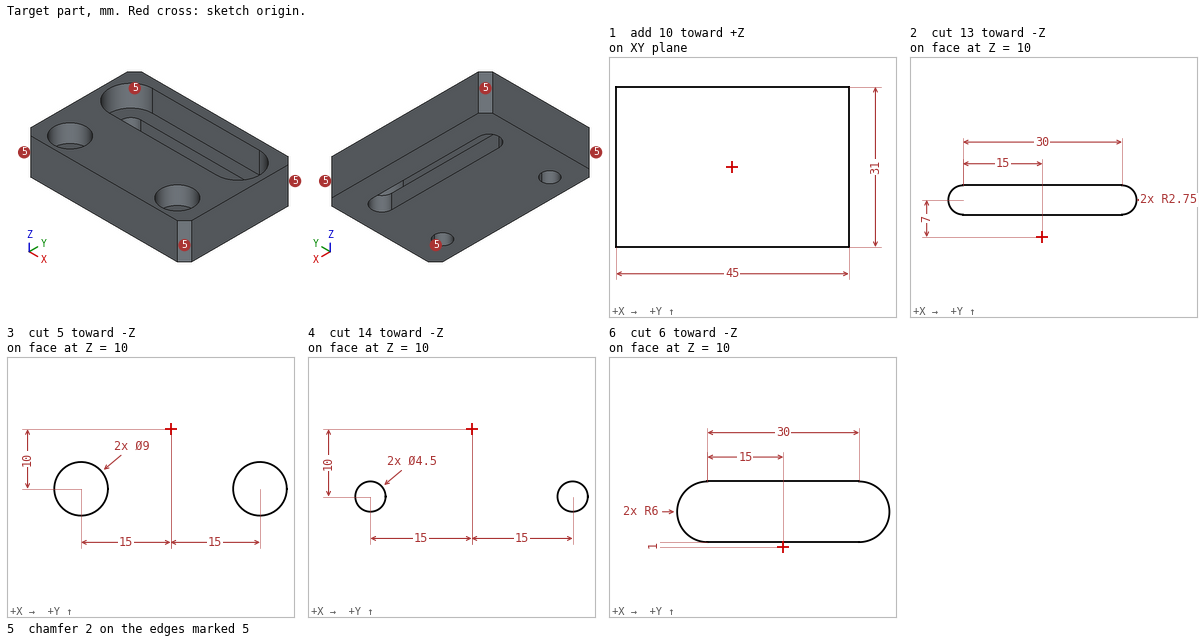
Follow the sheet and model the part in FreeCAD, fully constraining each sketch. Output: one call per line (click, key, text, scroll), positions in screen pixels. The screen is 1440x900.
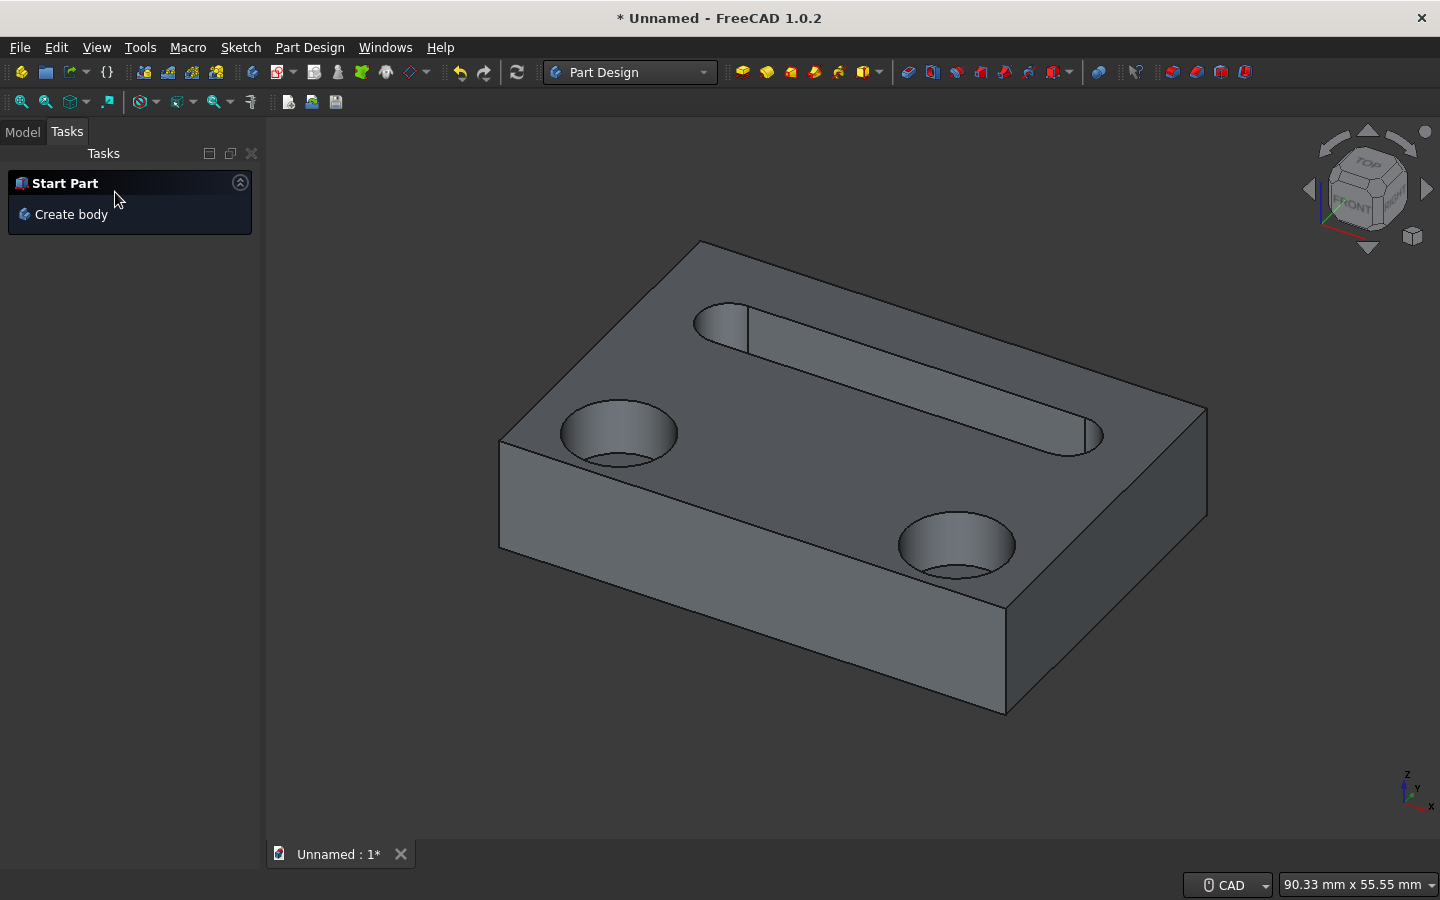
click(1006, 661)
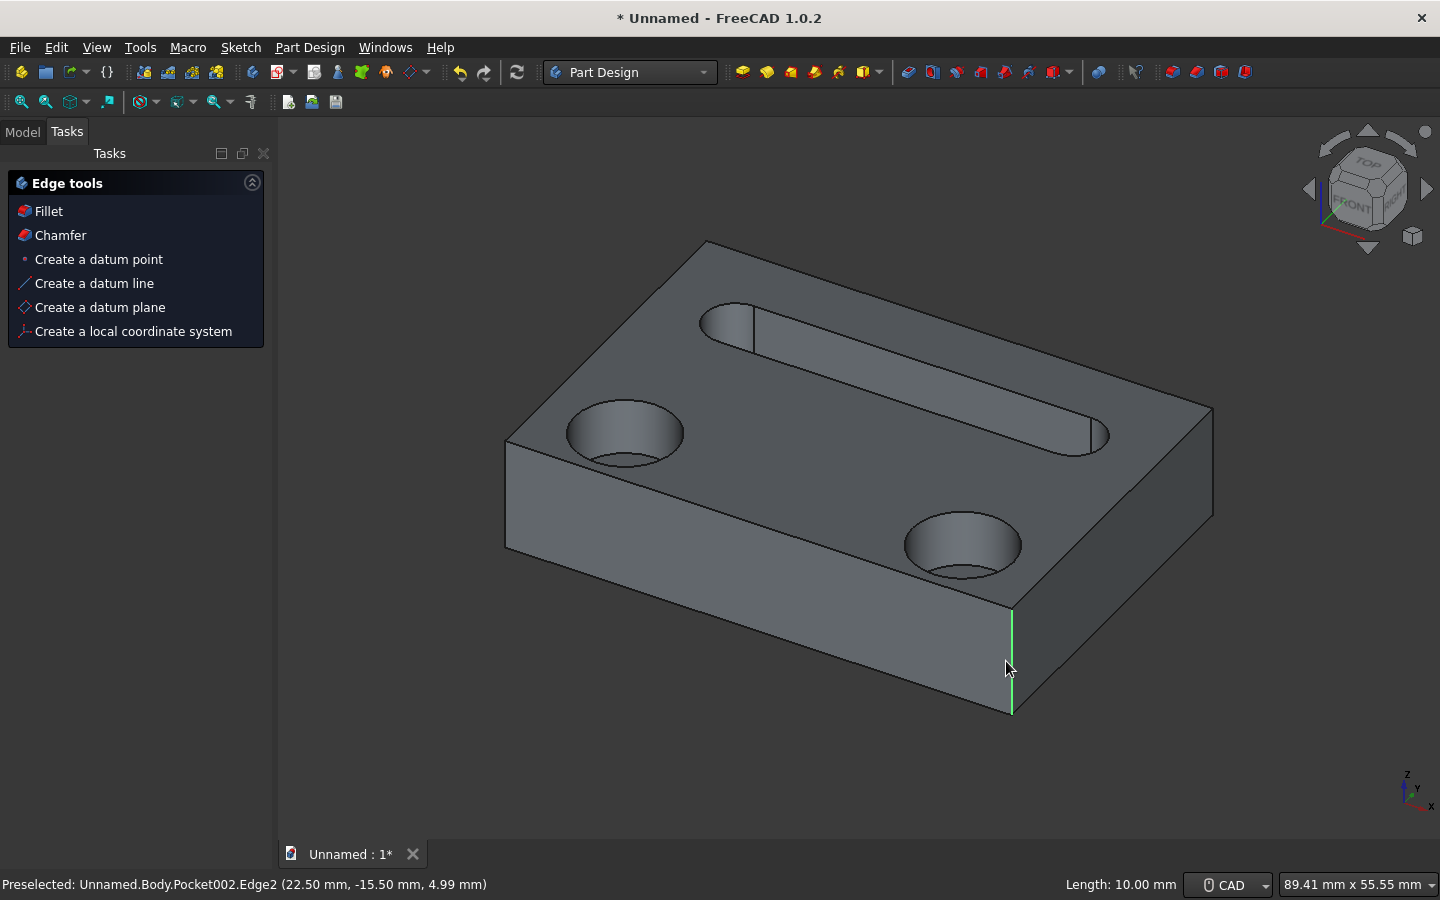
key(0)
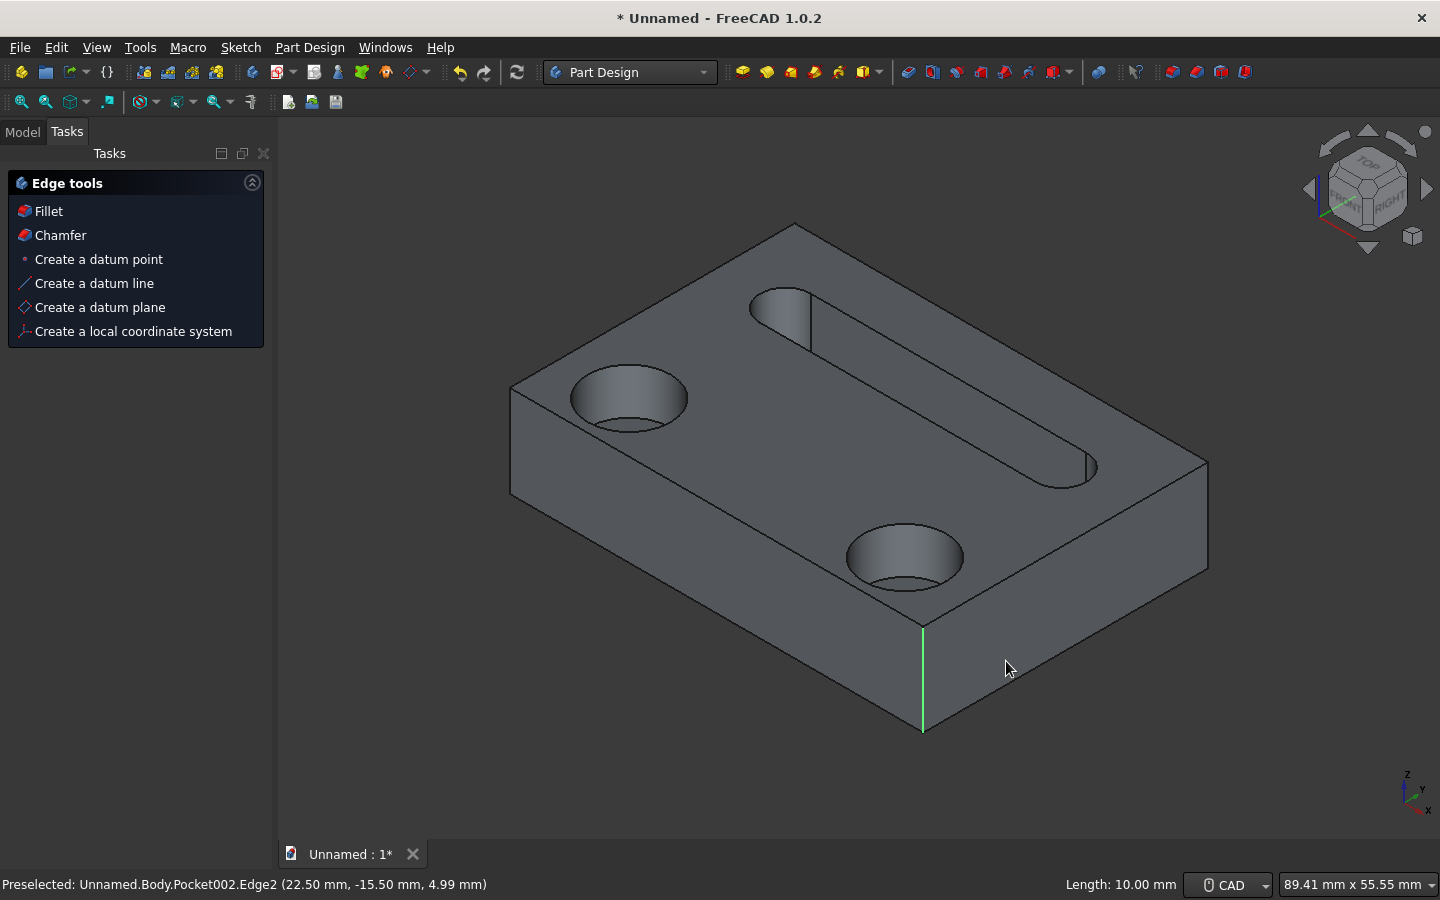
key(2)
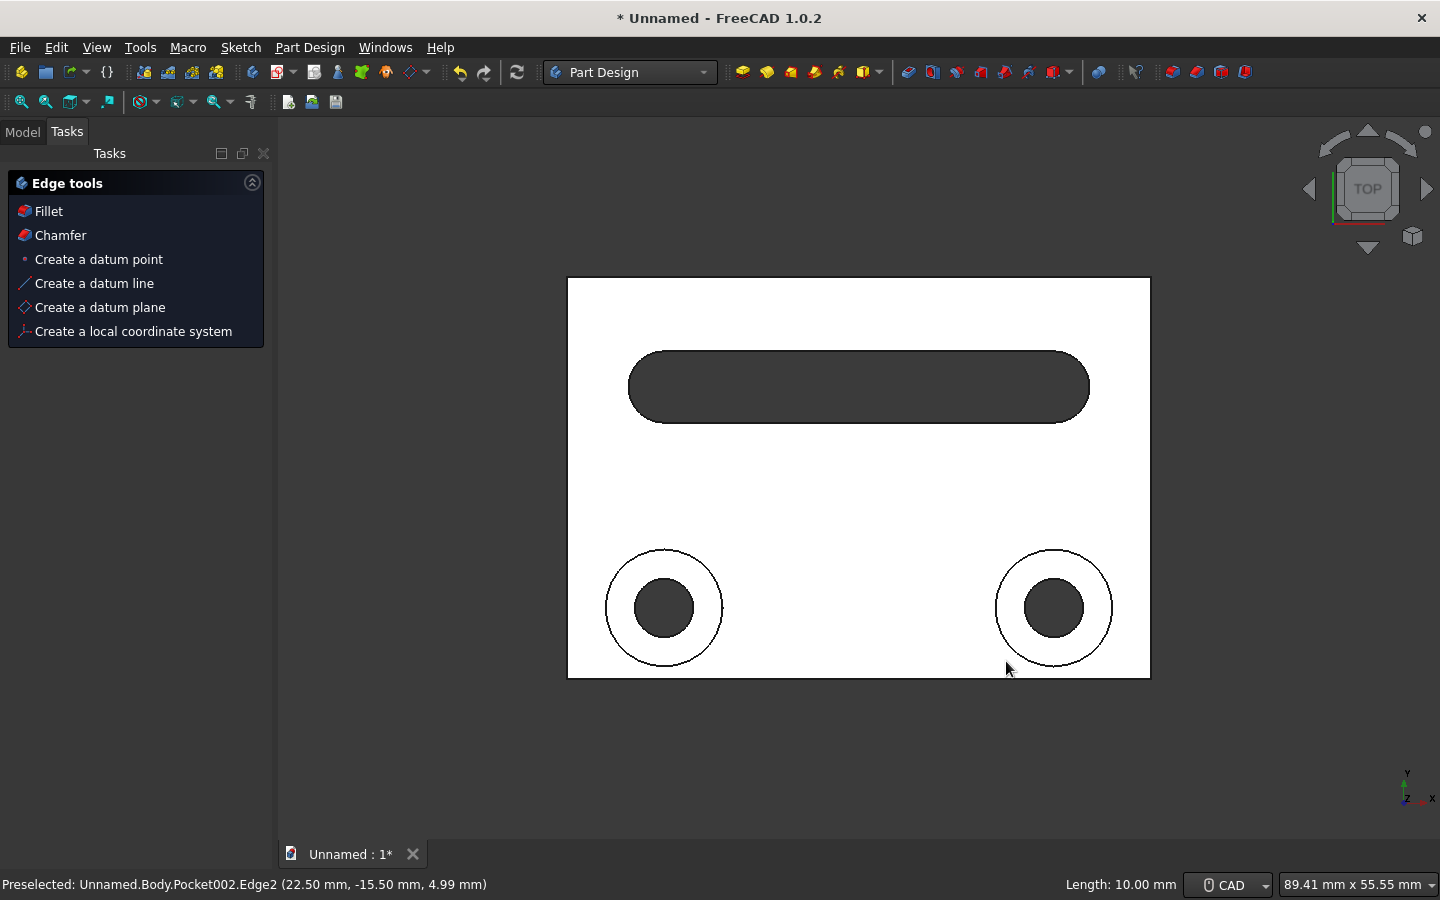
key(1)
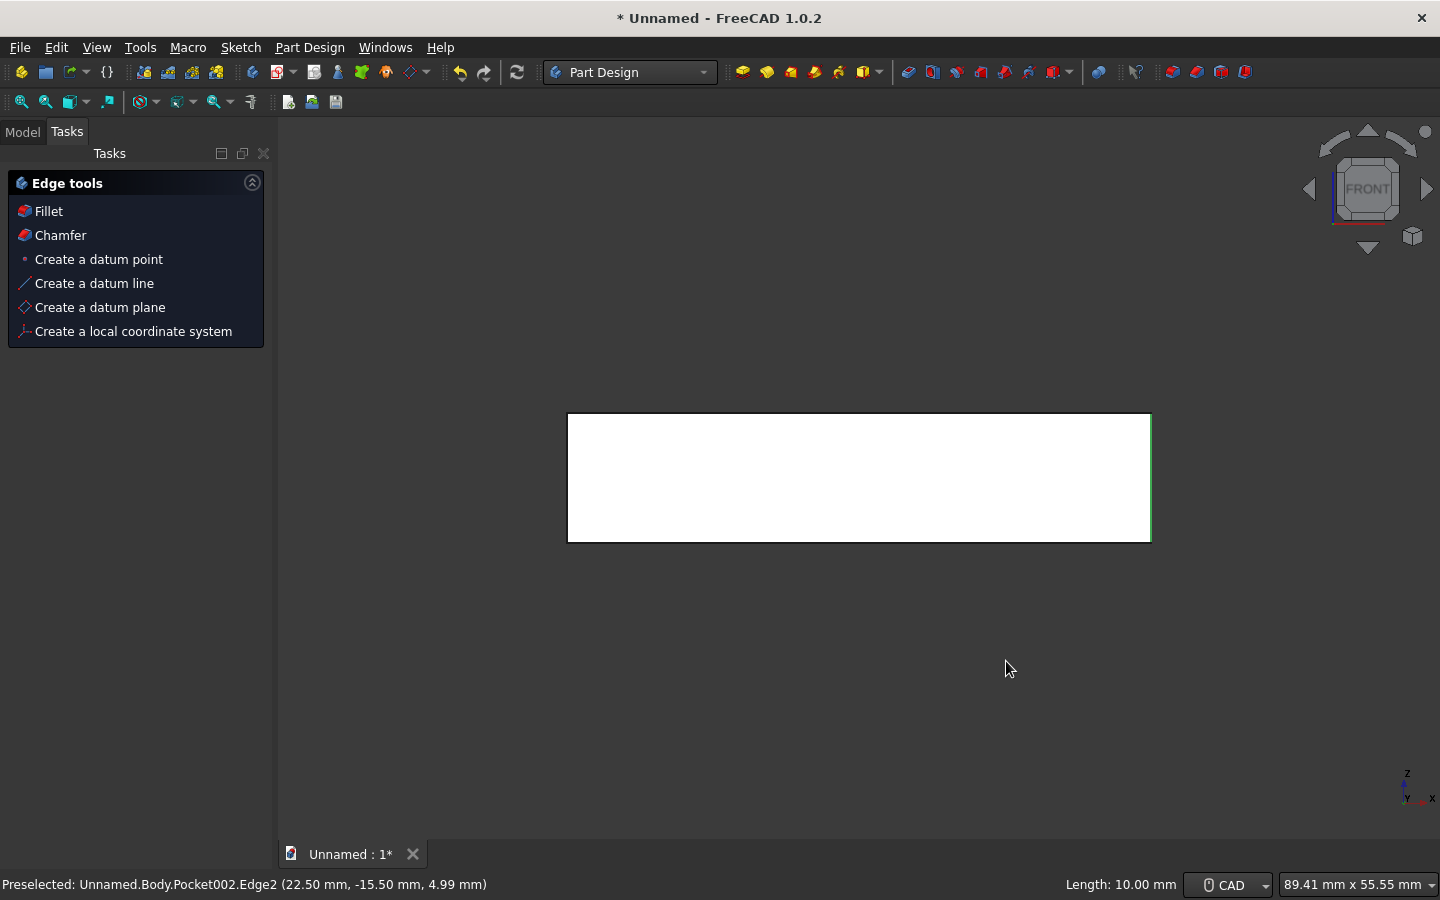
click(567, 477, ctrl)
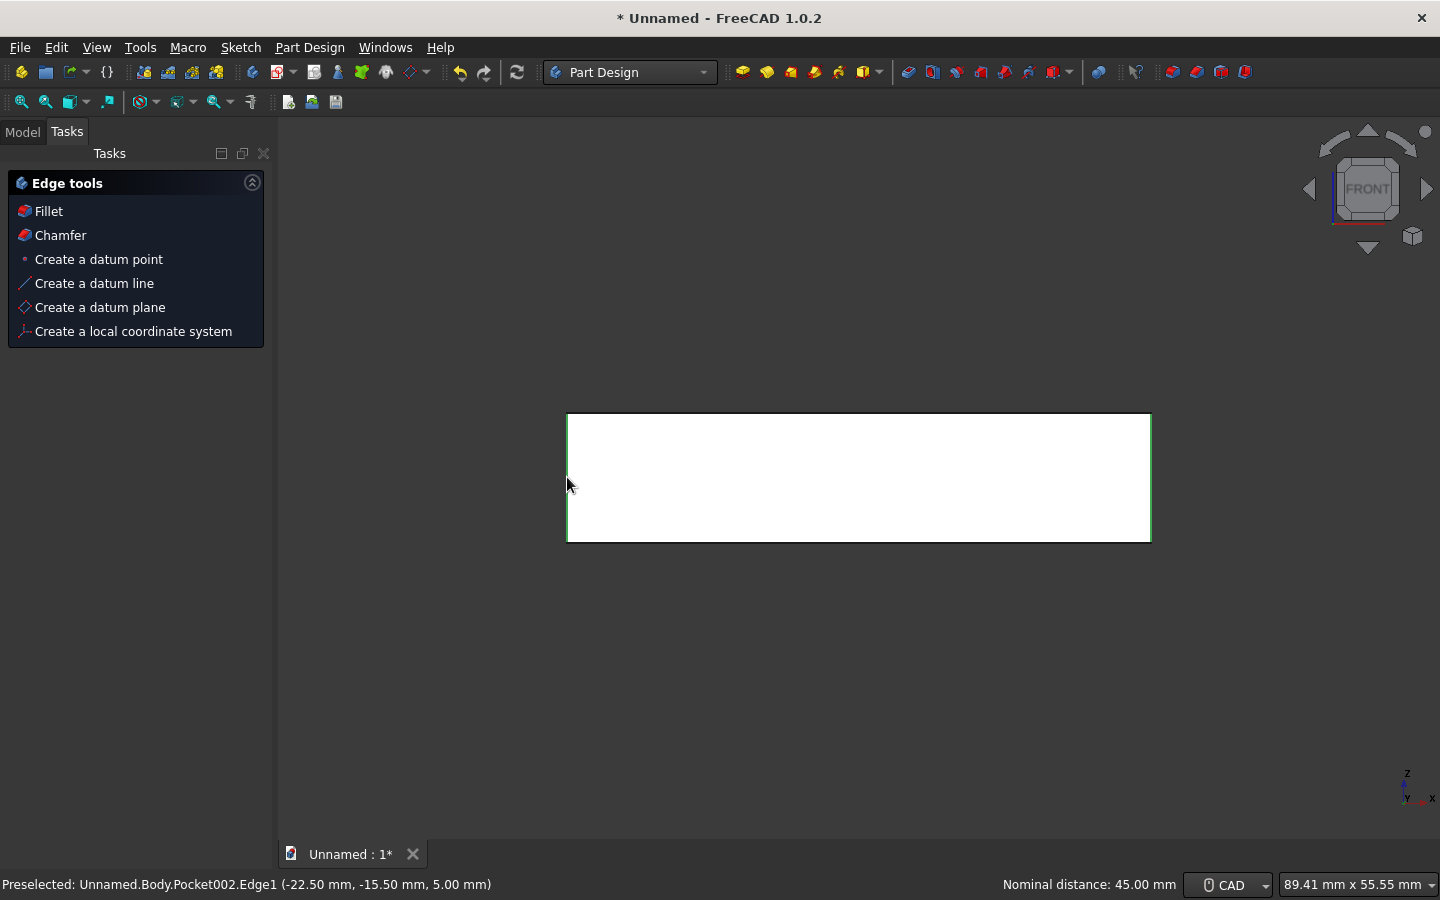
key(3)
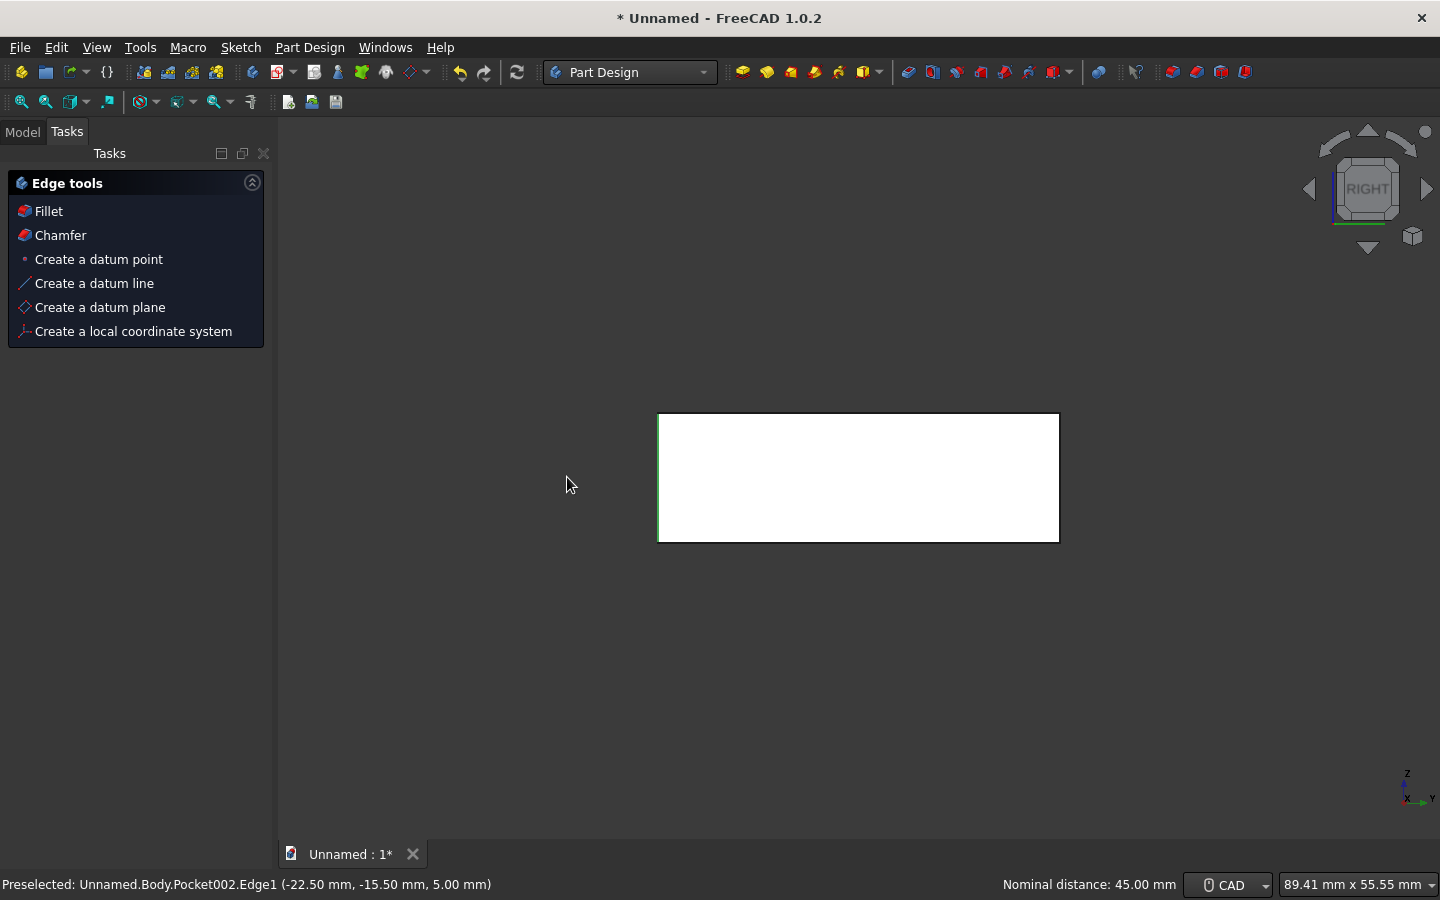
click(22, 102)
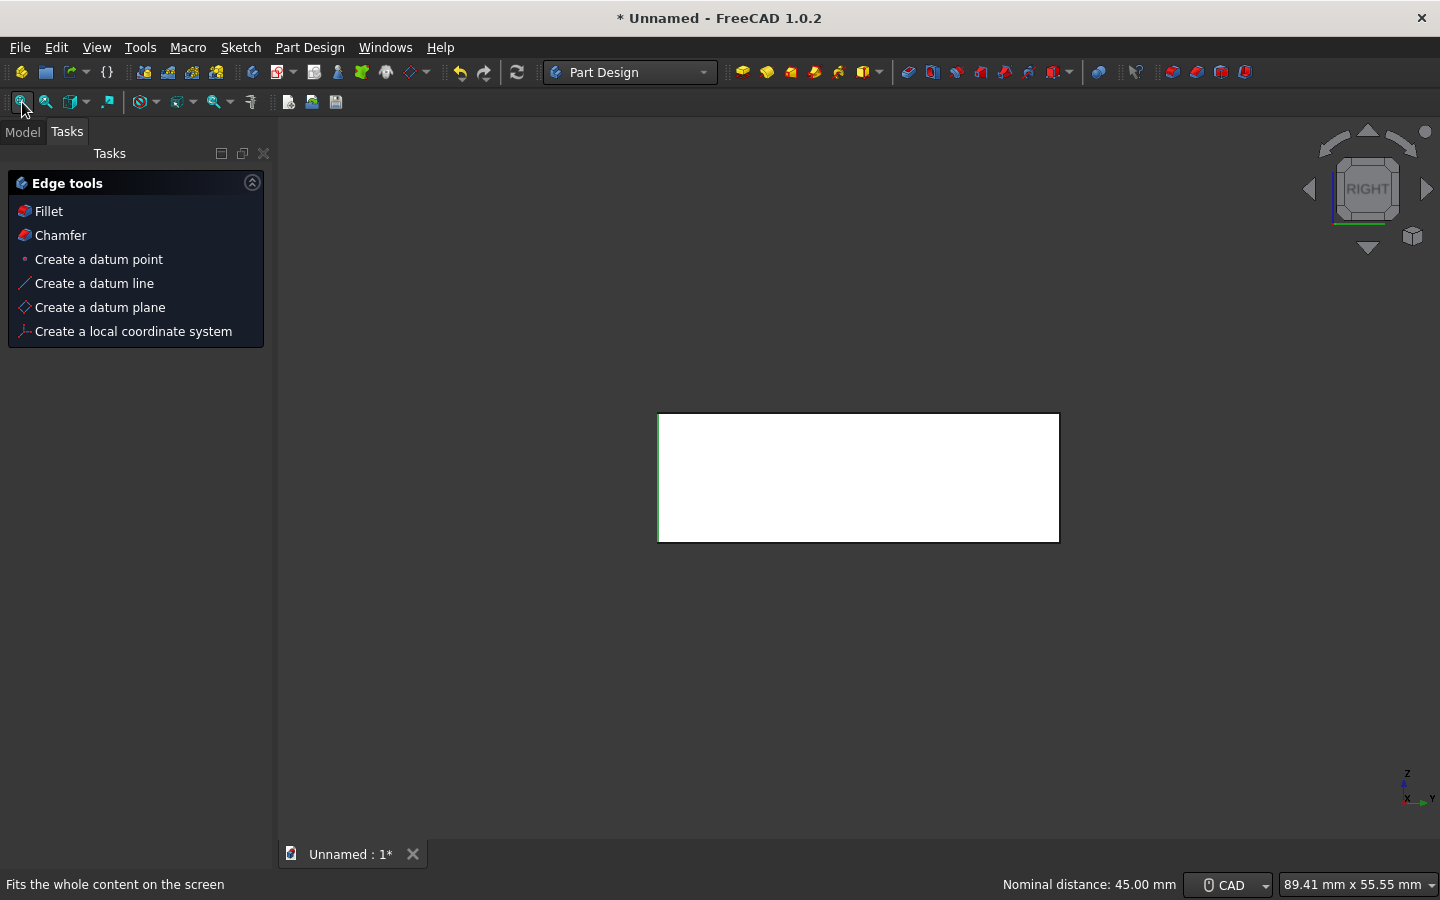
click(1060, 477, ctrl)